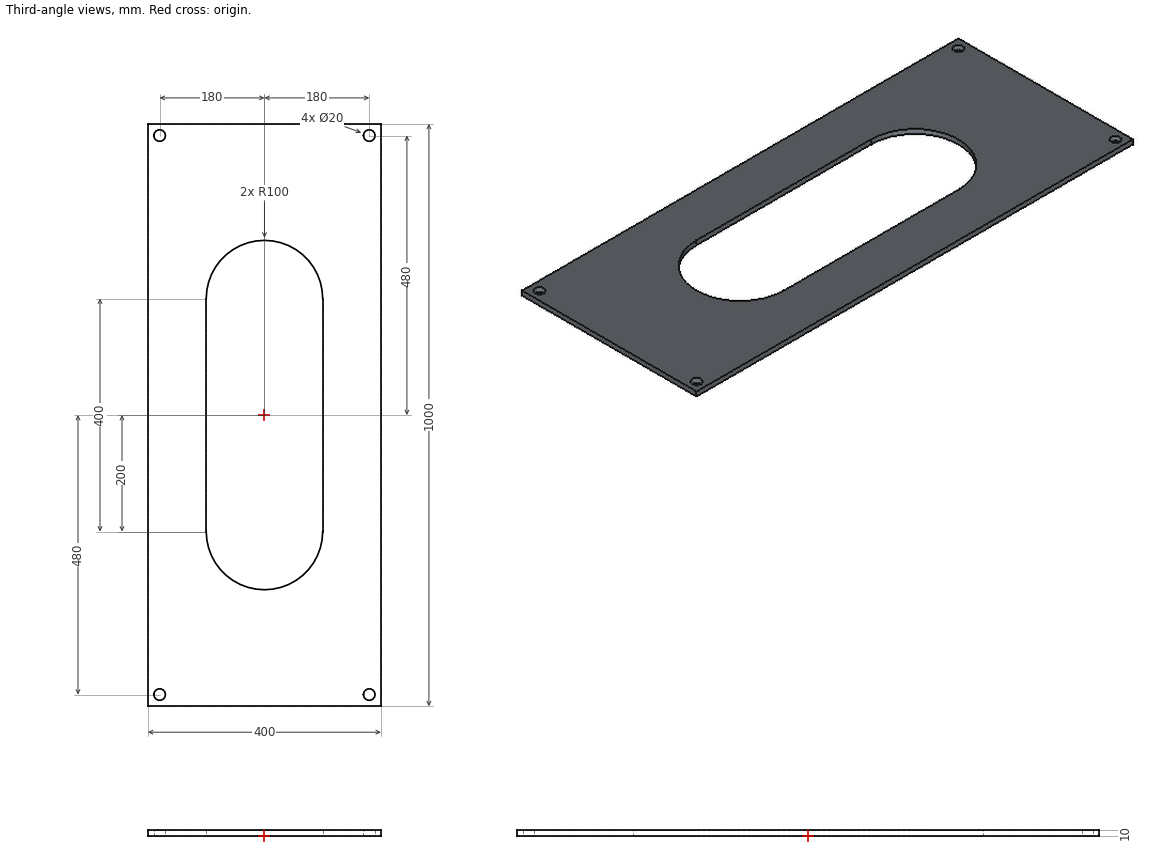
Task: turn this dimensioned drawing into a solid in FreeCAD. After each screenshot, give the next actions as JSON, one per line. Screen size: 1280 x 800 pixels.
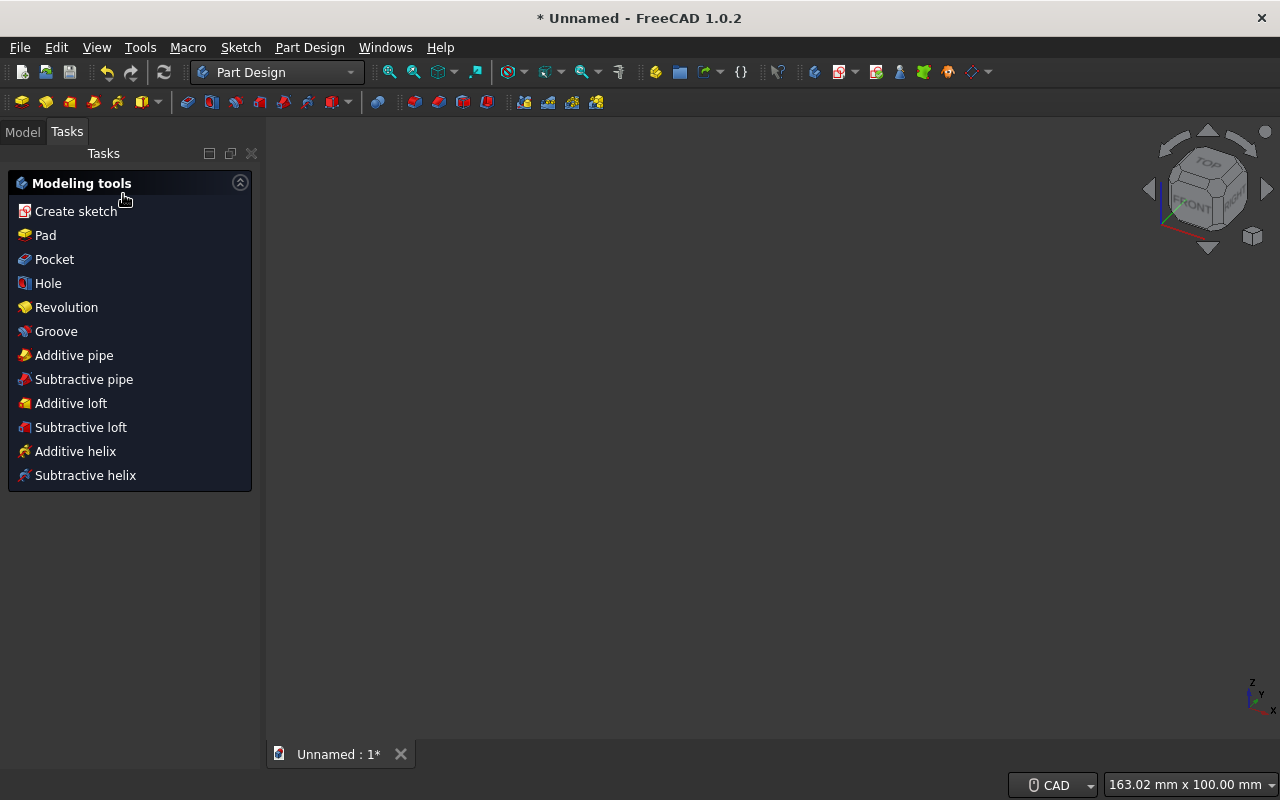
{"action": "left_click", "coordinate": [22, 102]}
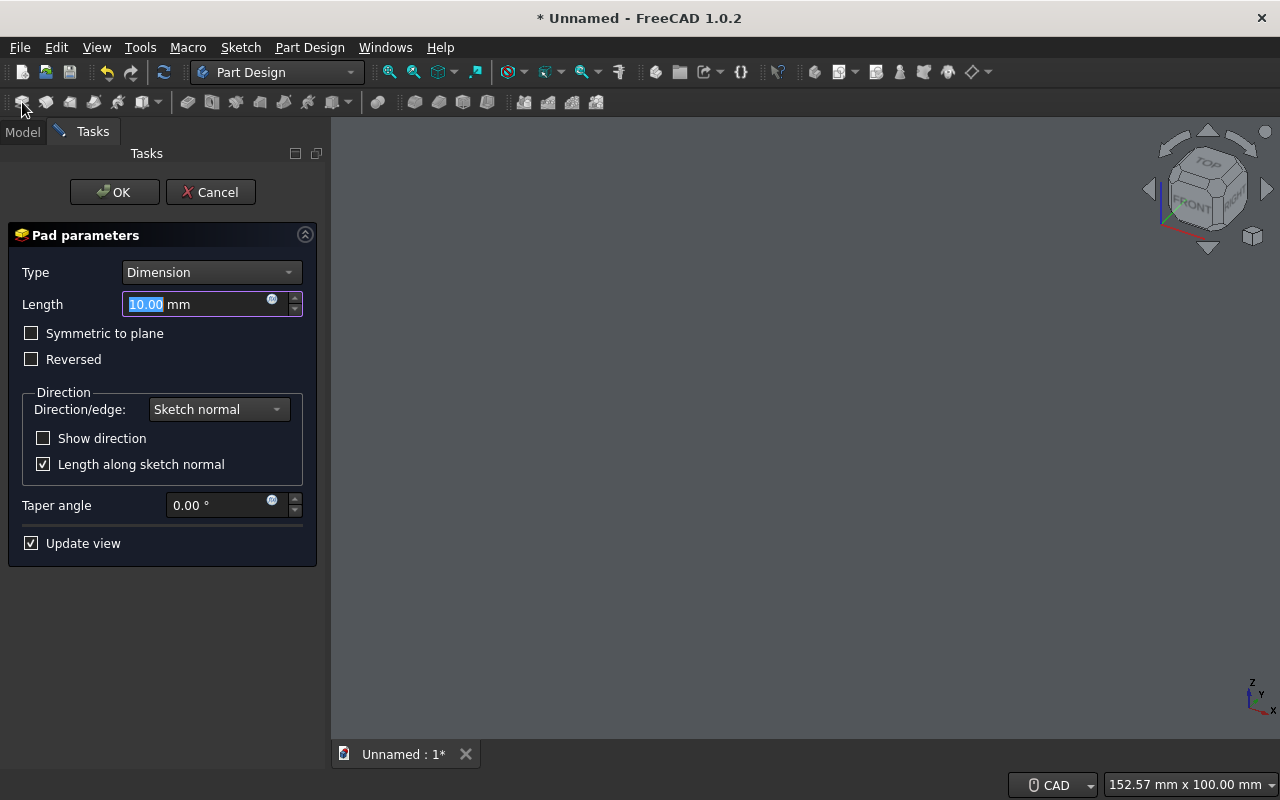
{"action": "type", "text": "10"}
{"action": "key", "text": "Tab"}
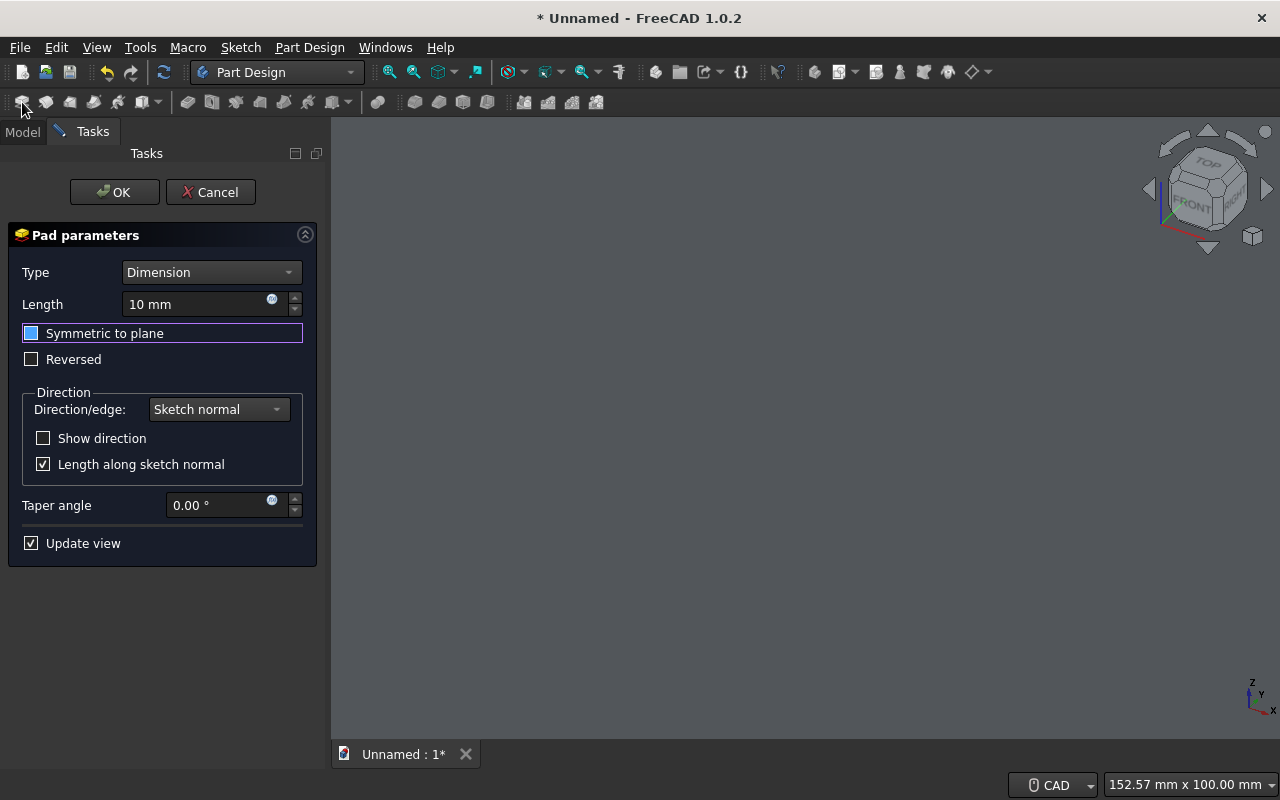
{"action": "left_click", "coordinate": [115, 192]}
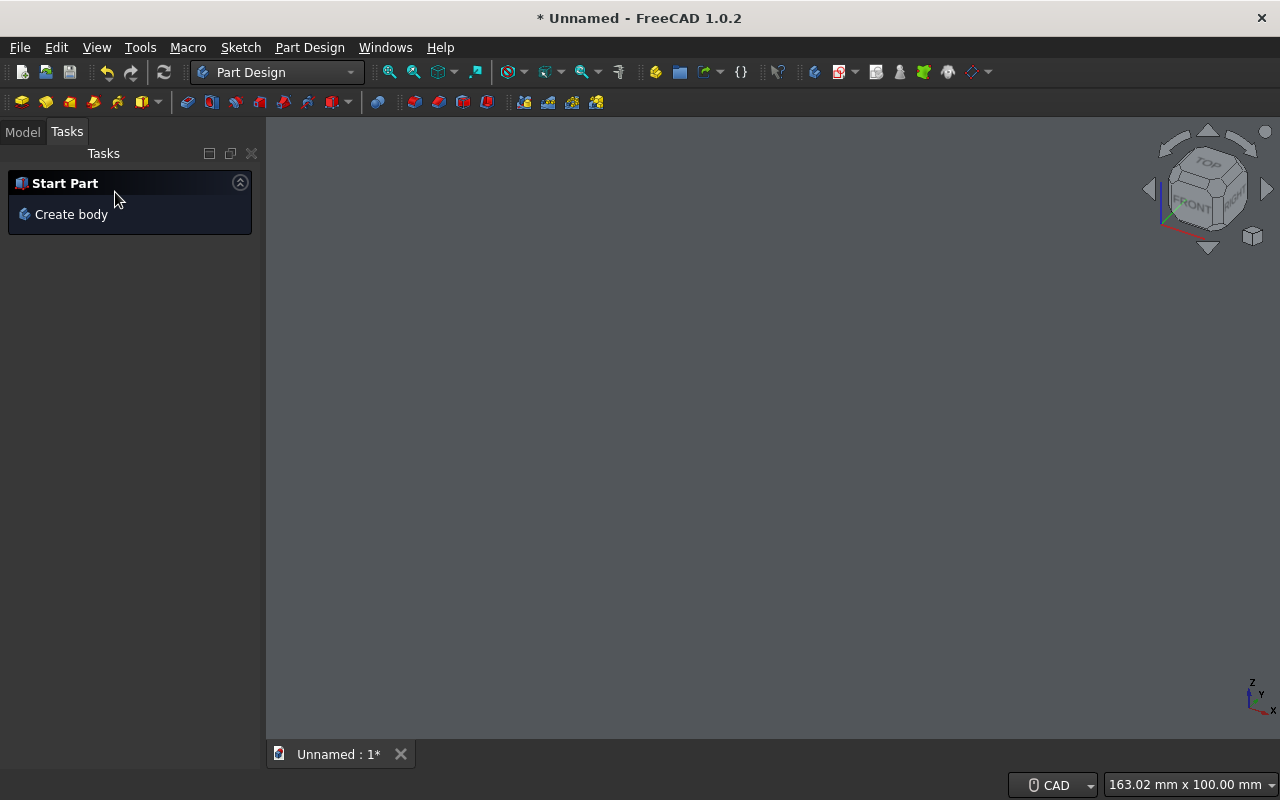
{"action": "left_click", "coordinate": [390, 72]}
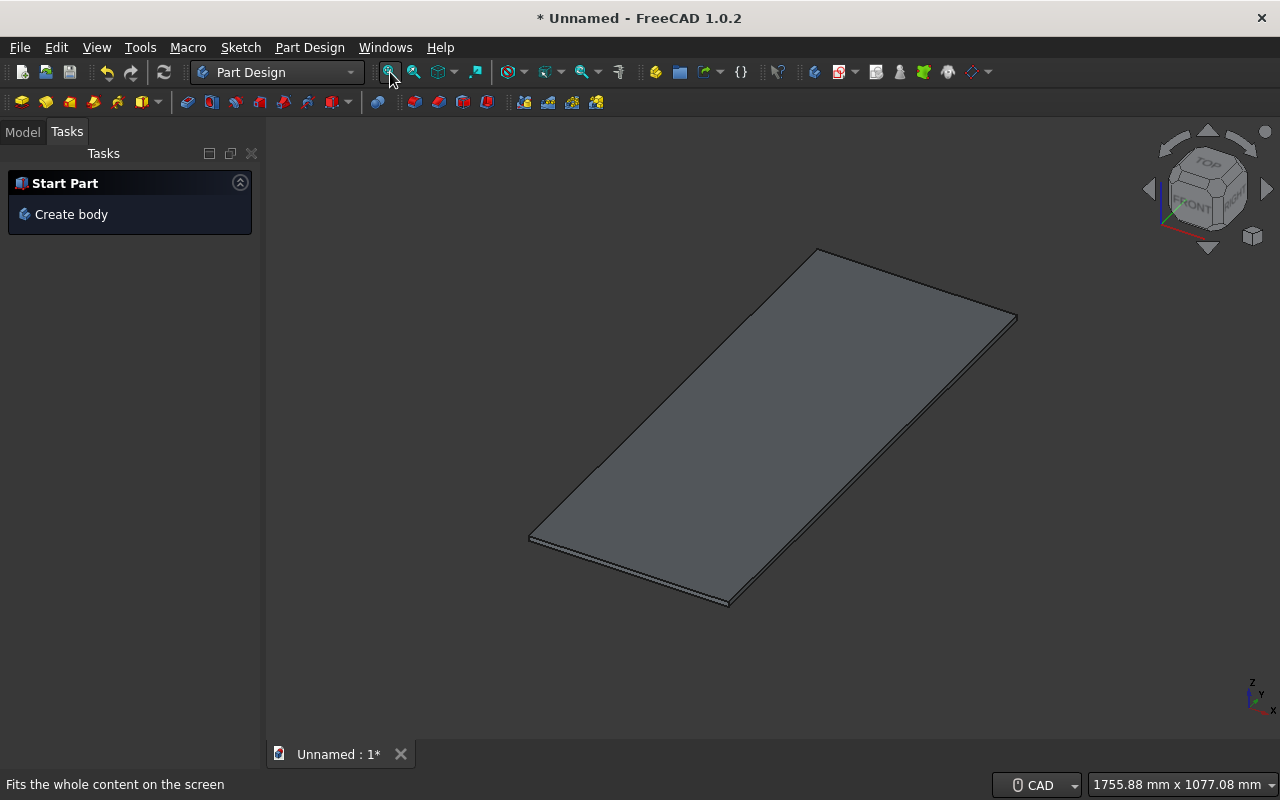
{"action": "left_click", "coordinate": [840, 72]}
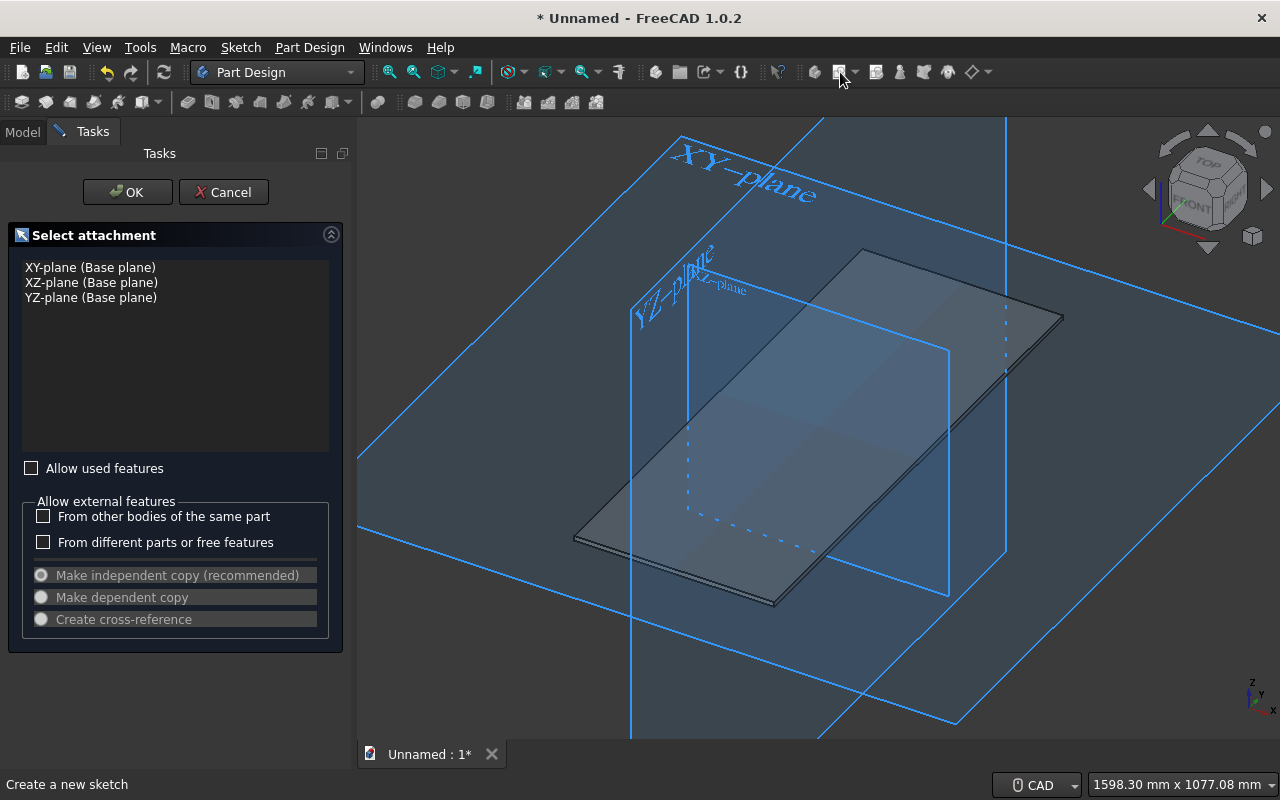
{"action": "left_click", "coordinate": [82, 268]}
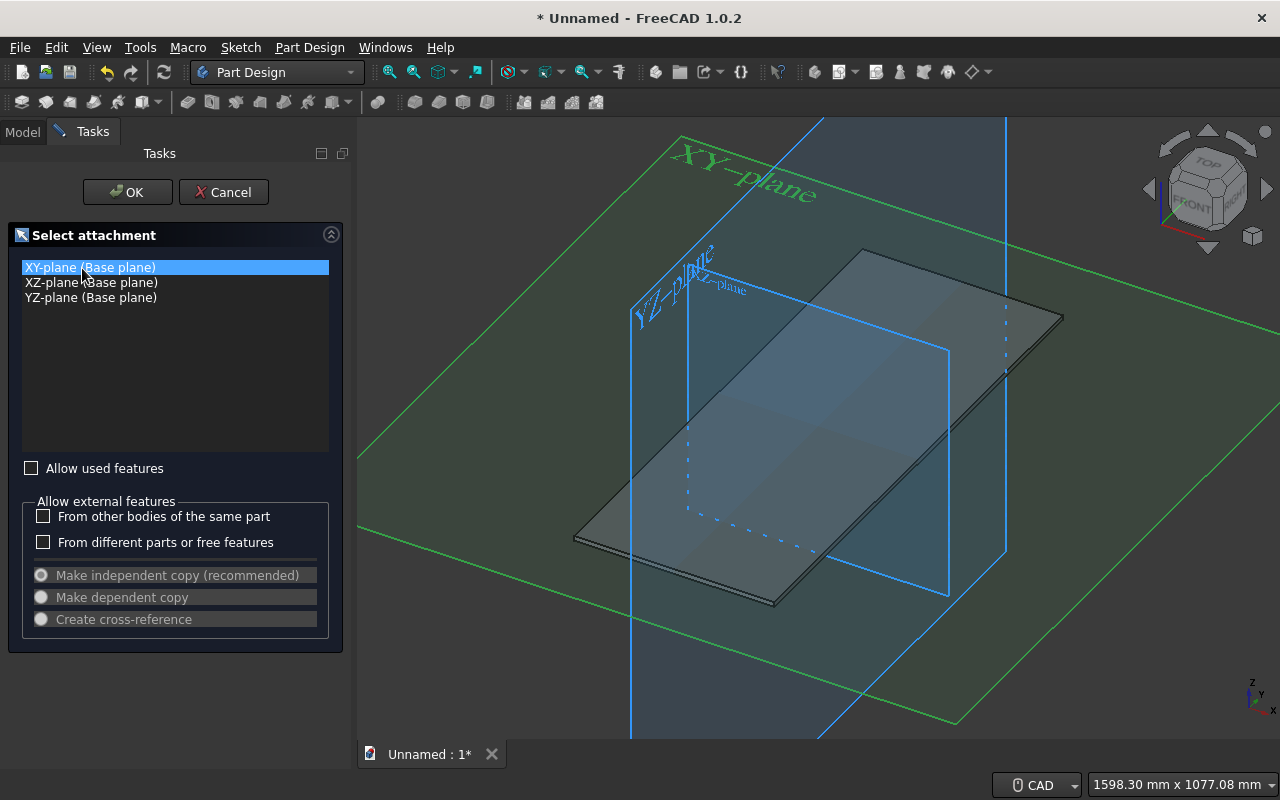
{"action": "left_click", "coordinate": [128, 192]}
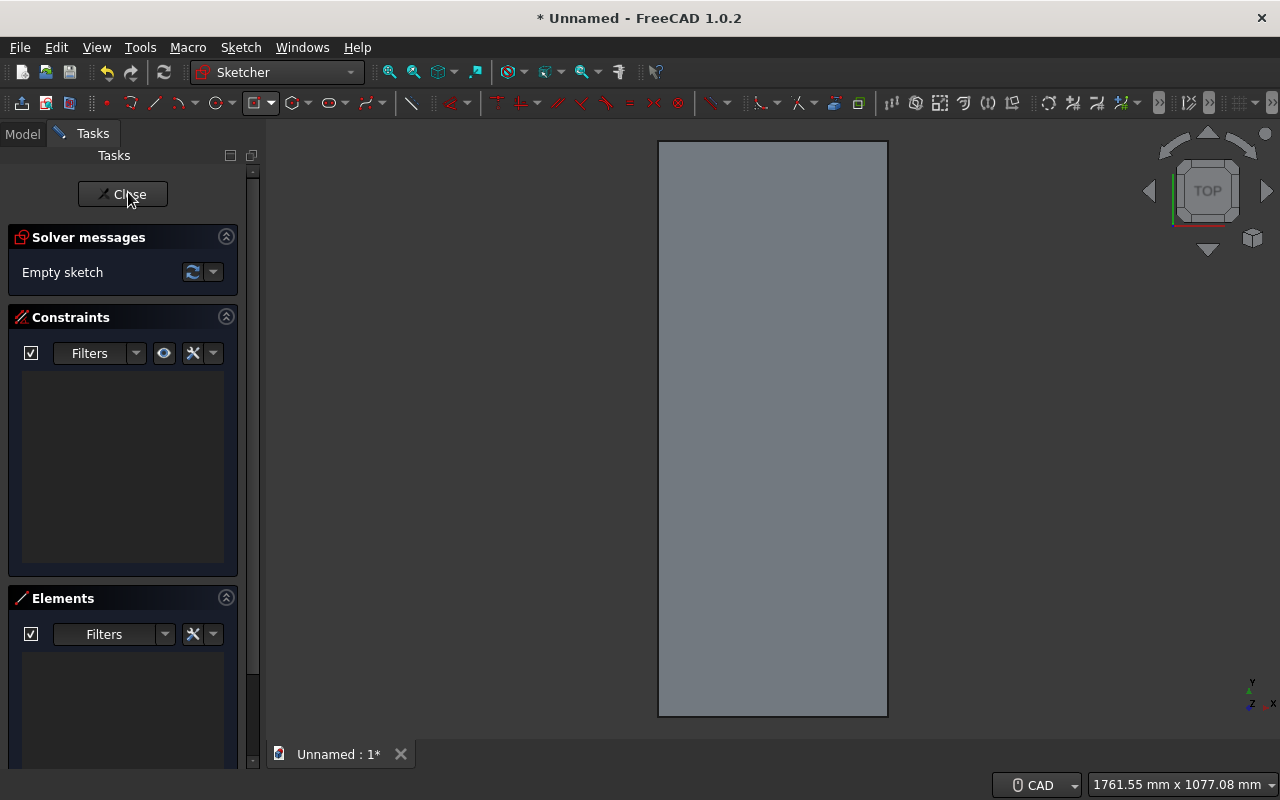
{"action": "left_click", "coordinate": [70, 104]}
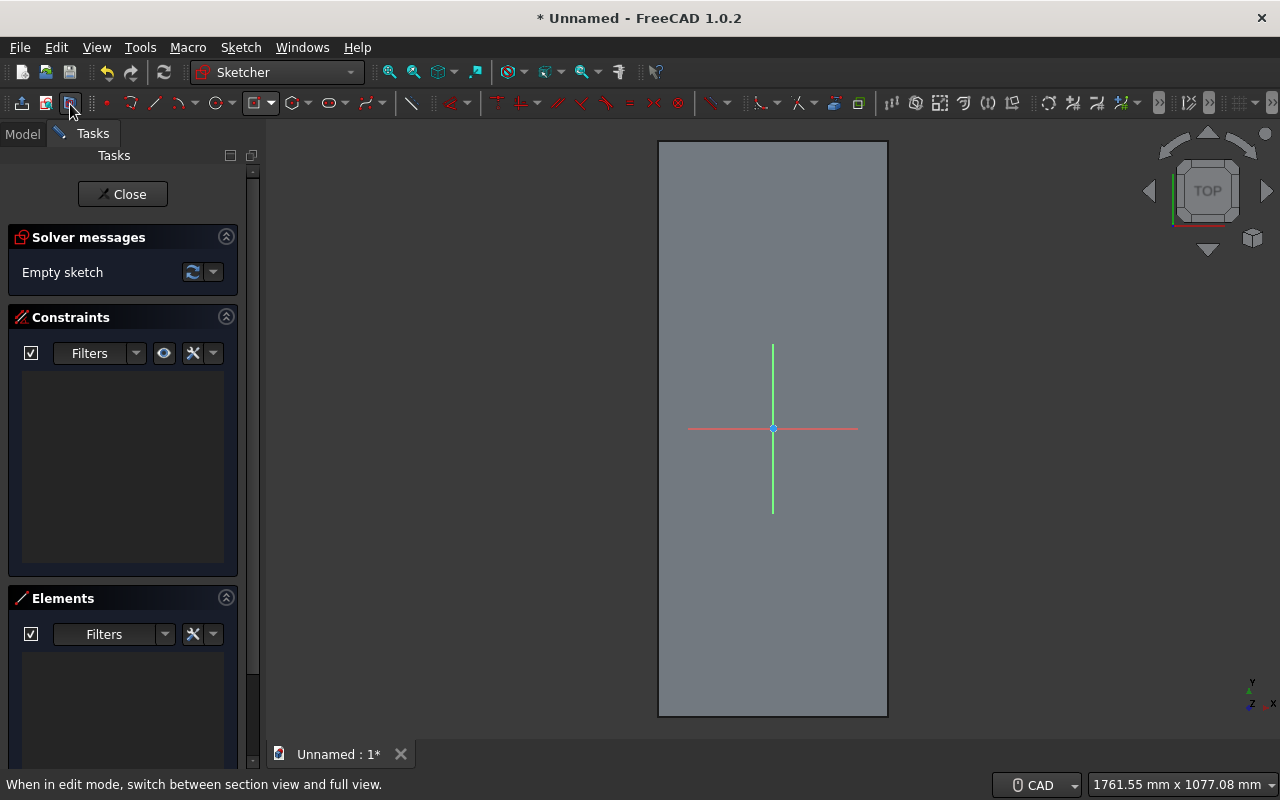
{"action": "scroll", "coordinate": [565, 429], "scroll_direction": "down", "scroll_amount": 2}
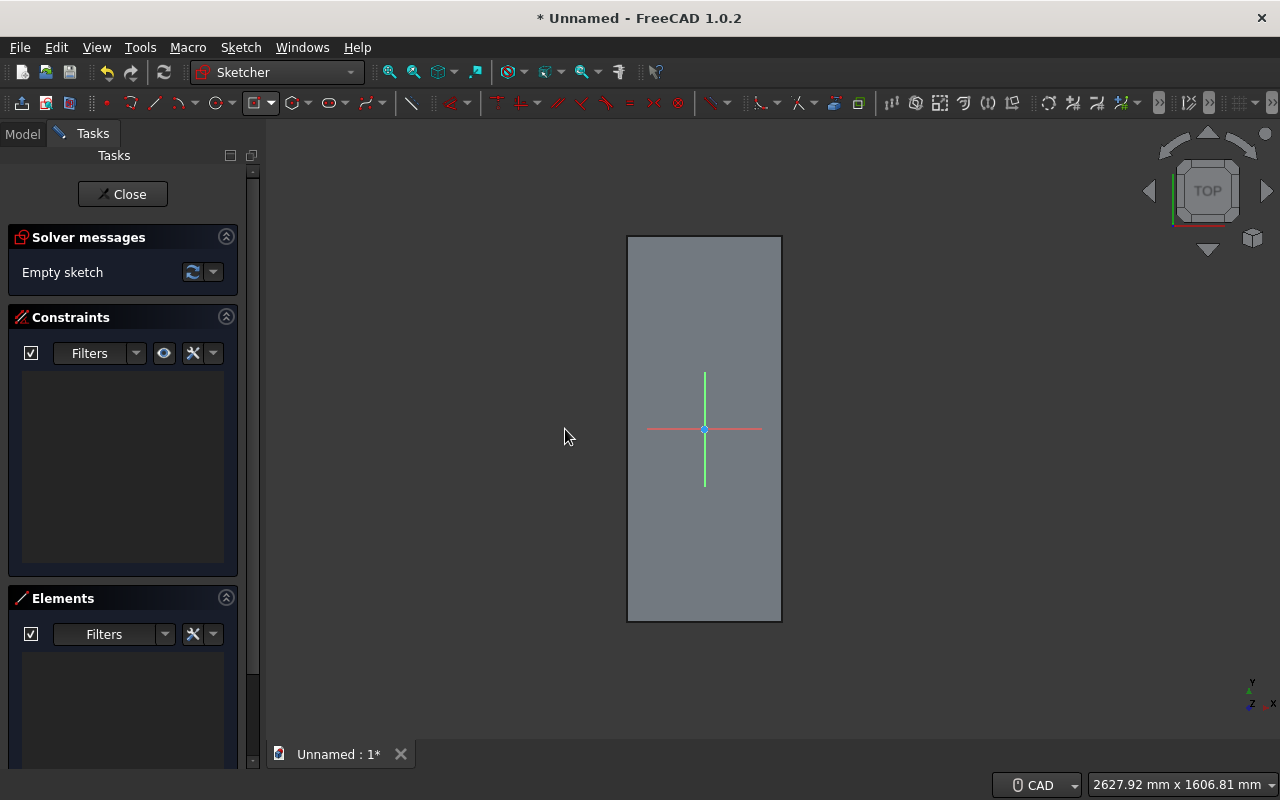
{"action": "left_click", "coordinate": [216, 104]}